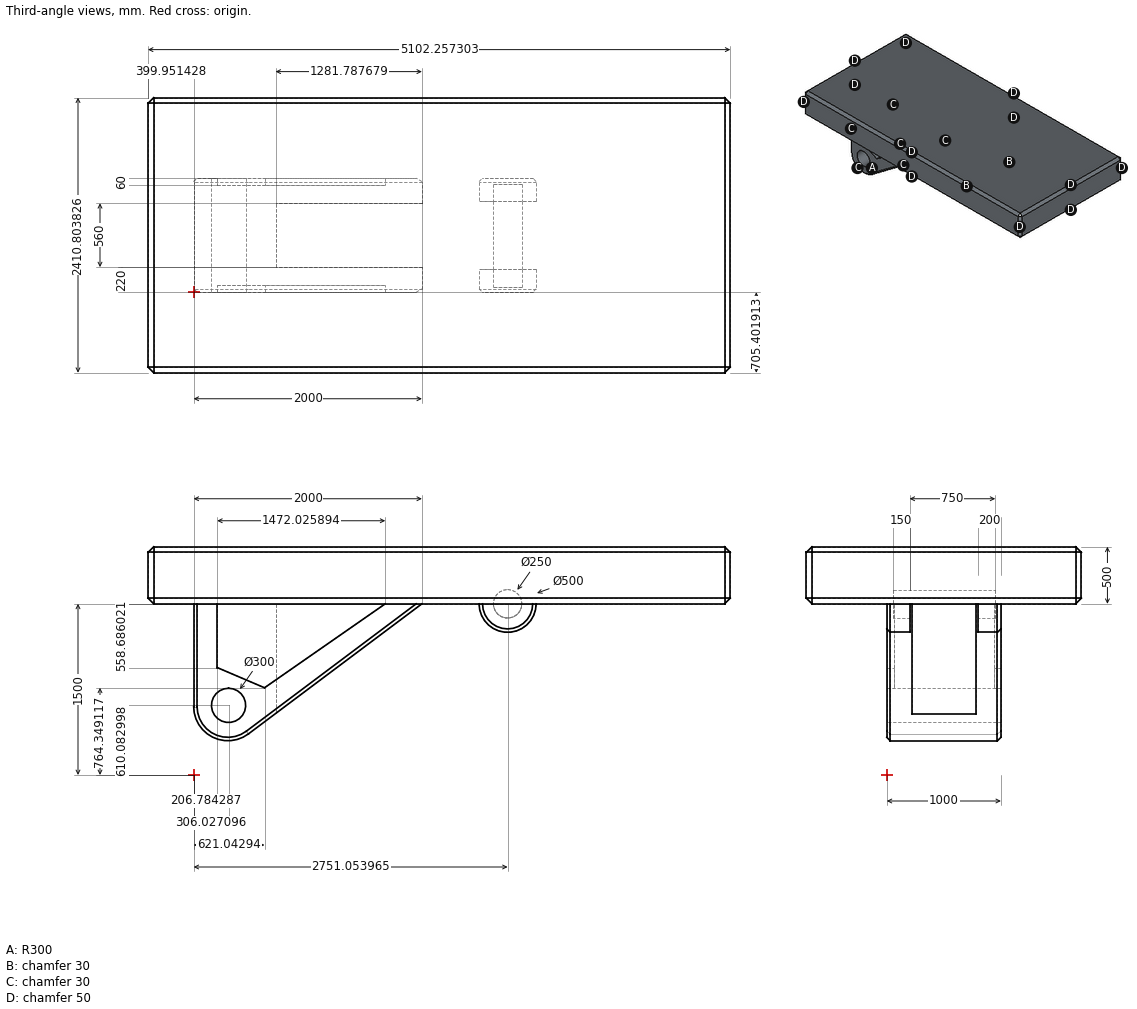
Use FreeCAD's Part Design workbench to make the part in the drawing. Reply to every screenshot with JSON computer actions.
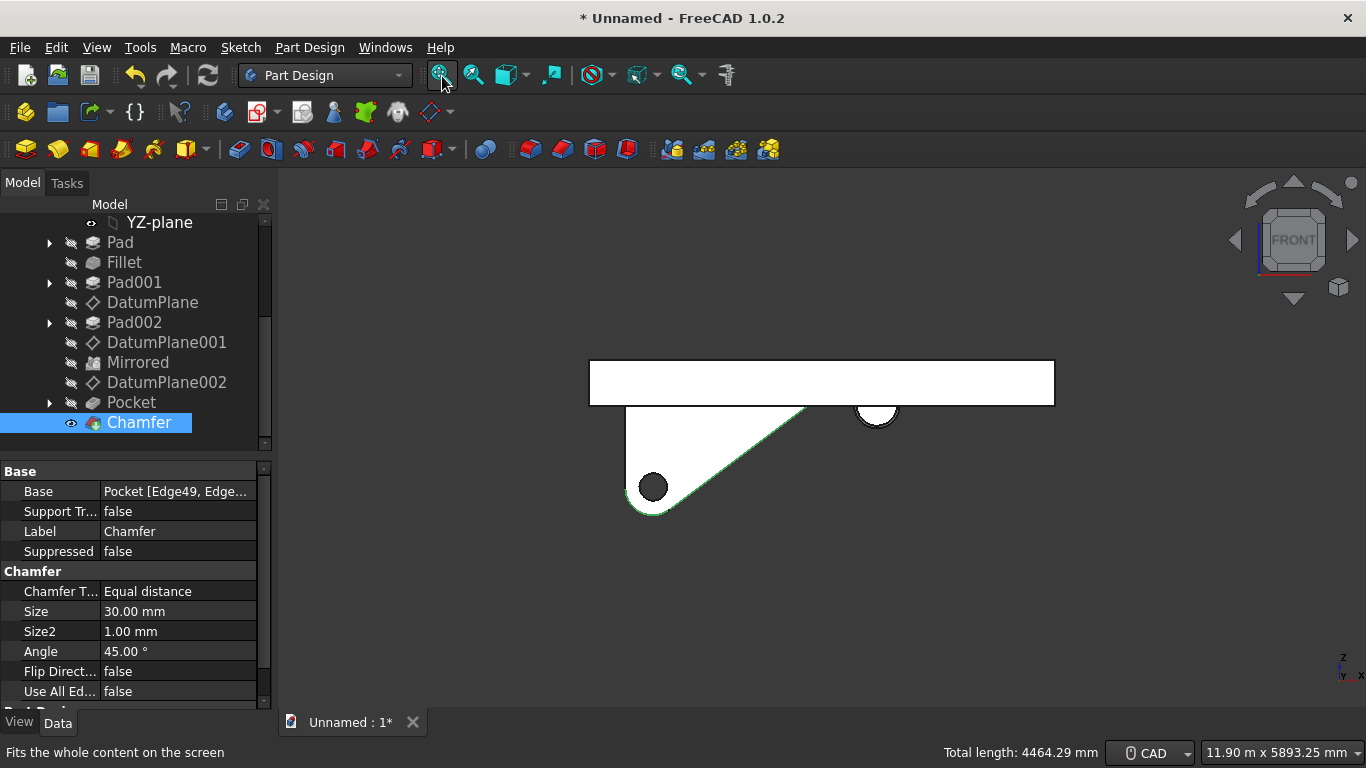
{"action": "left_click", "coordinate": [442, 76]}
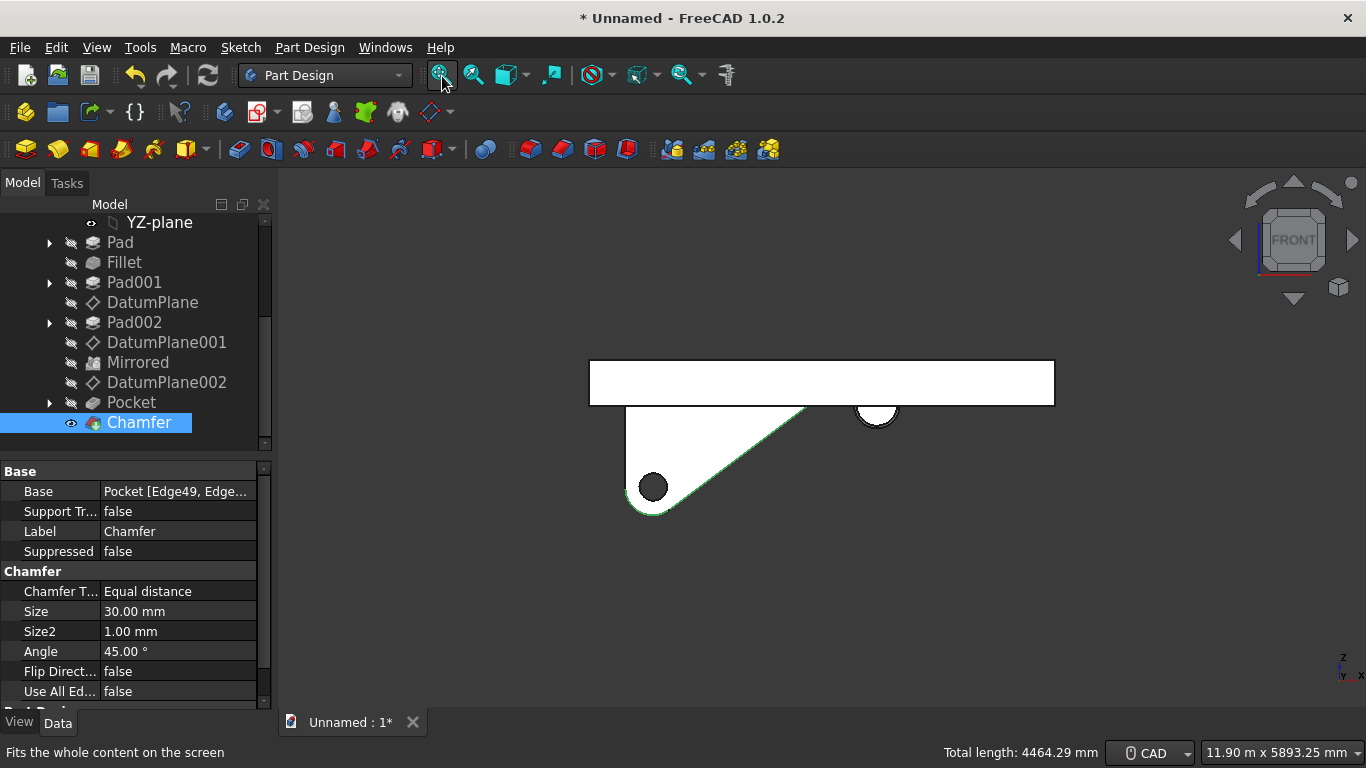
{"action": "left_click", "coordinate": [625, 446], "text": "ctrl"}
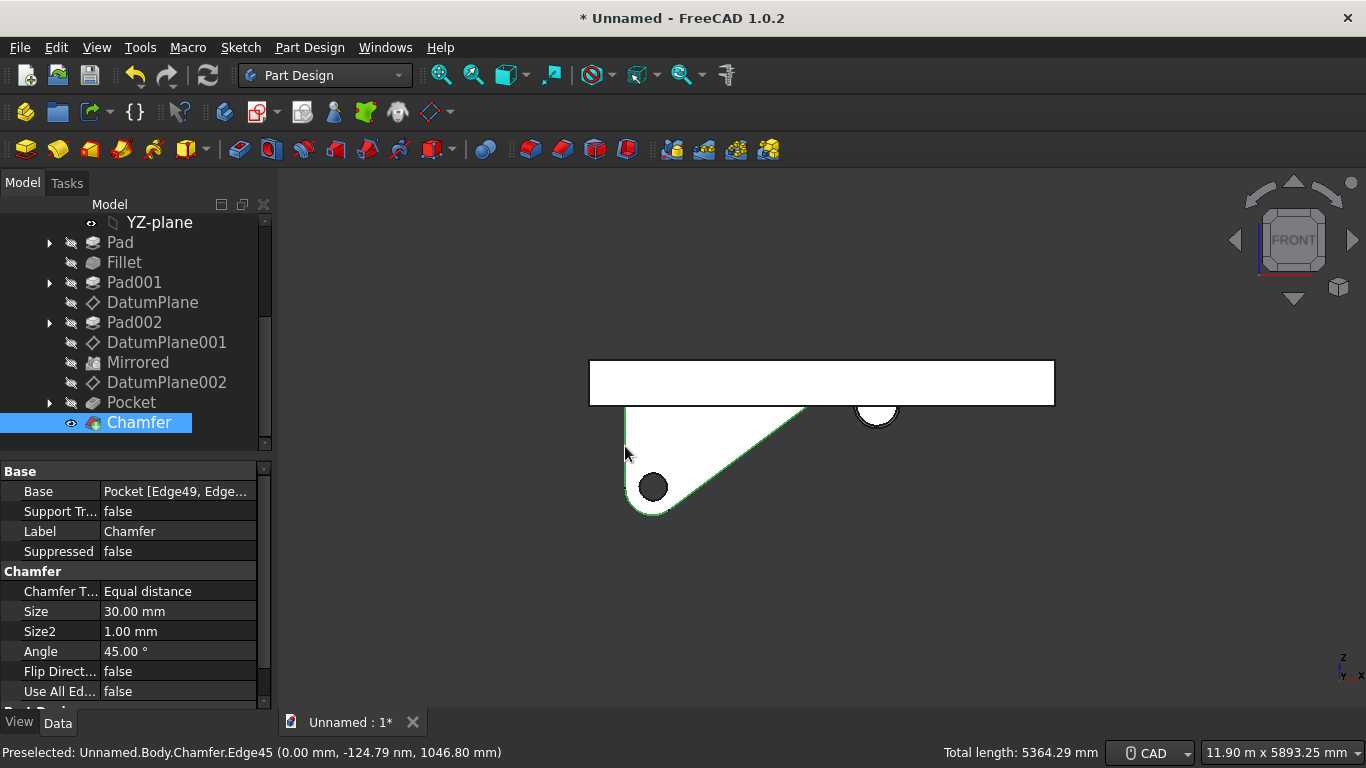
{"action": "key", "text": "3"}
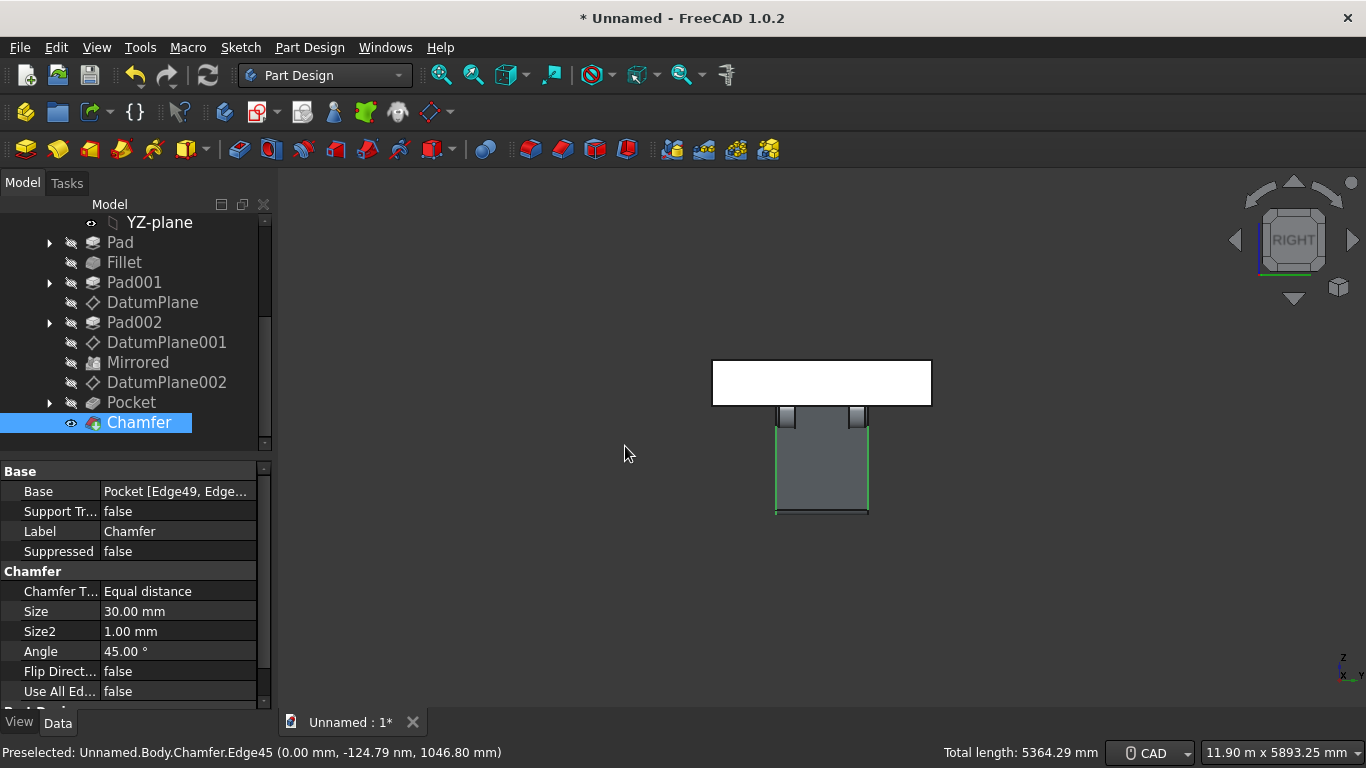
{"action": "left_click", "coordinate": [442, 76]}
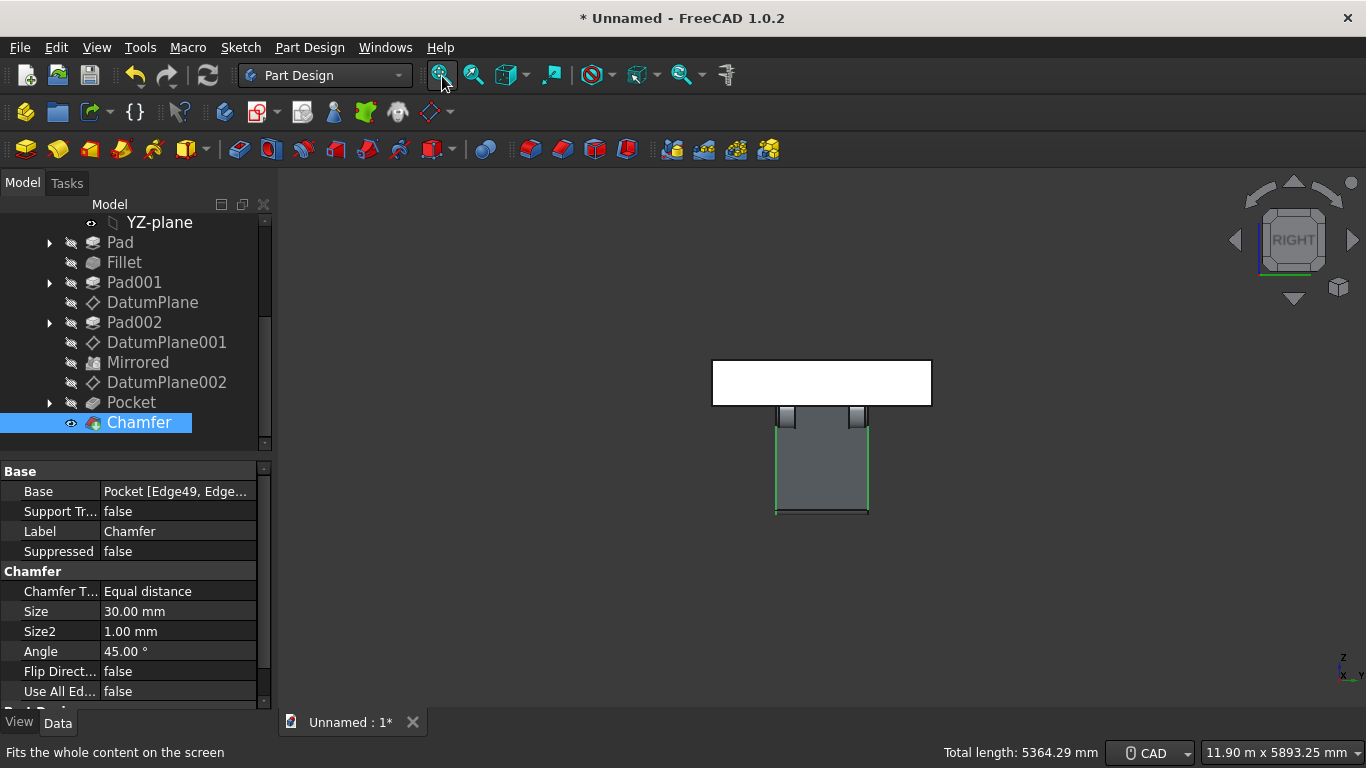
{"action": "key", "text": "5"}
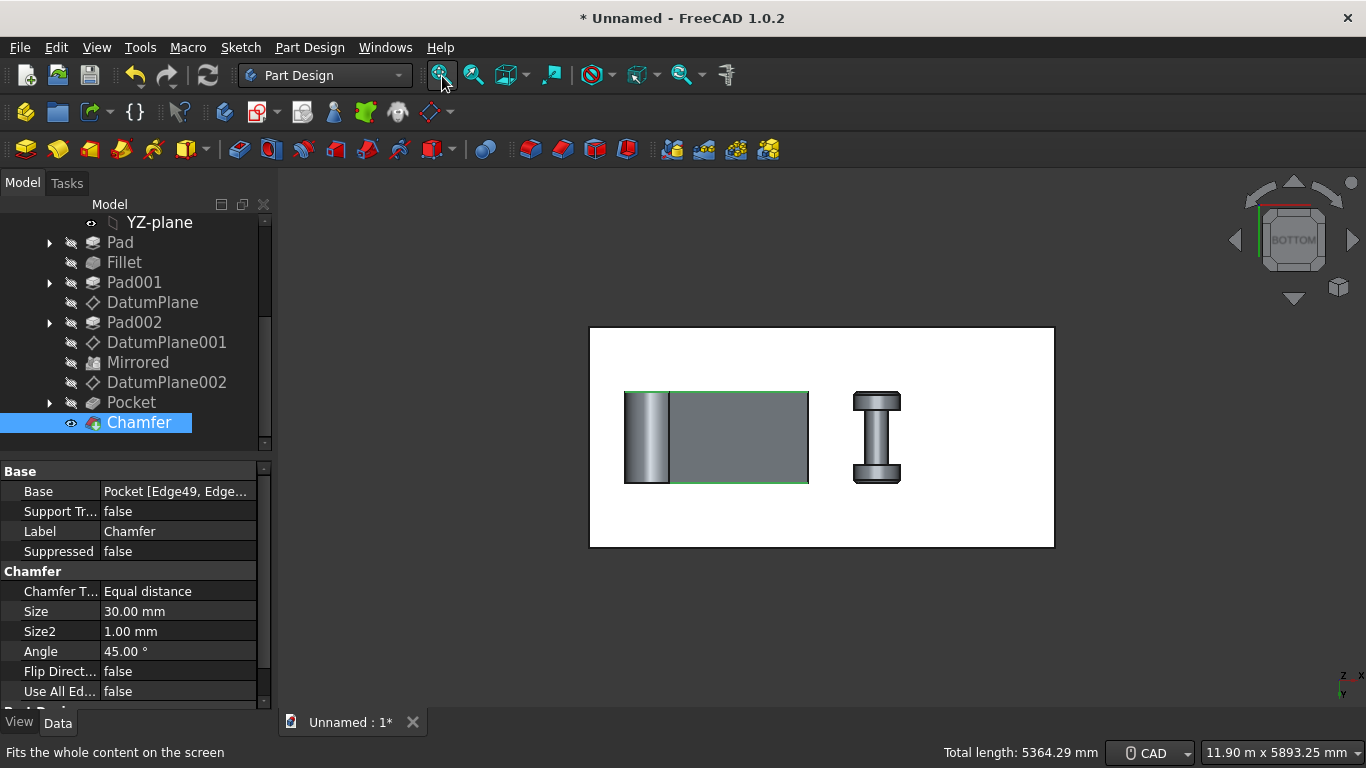
{"action": "key", "text": "v f"}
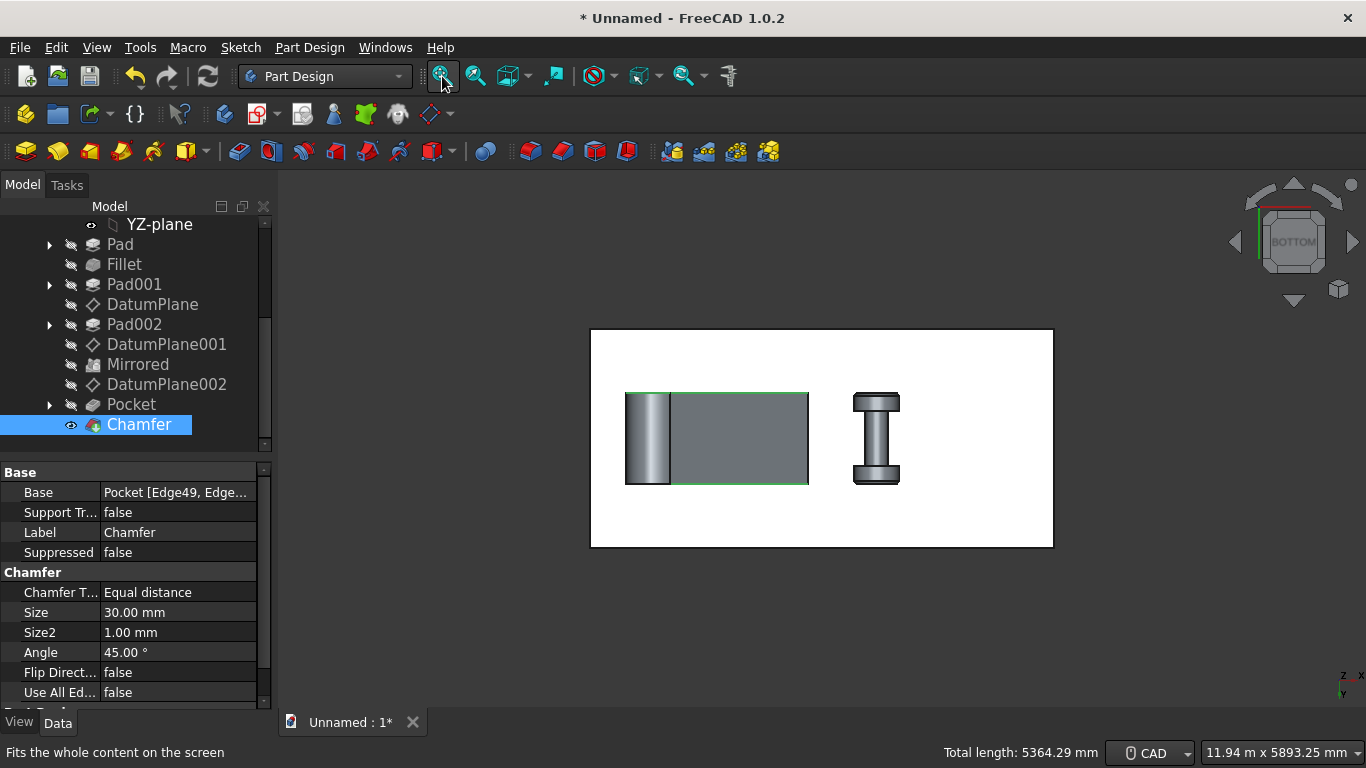
{"action": "left_click", "coordinate": [641, 483], "text": "ctrl"}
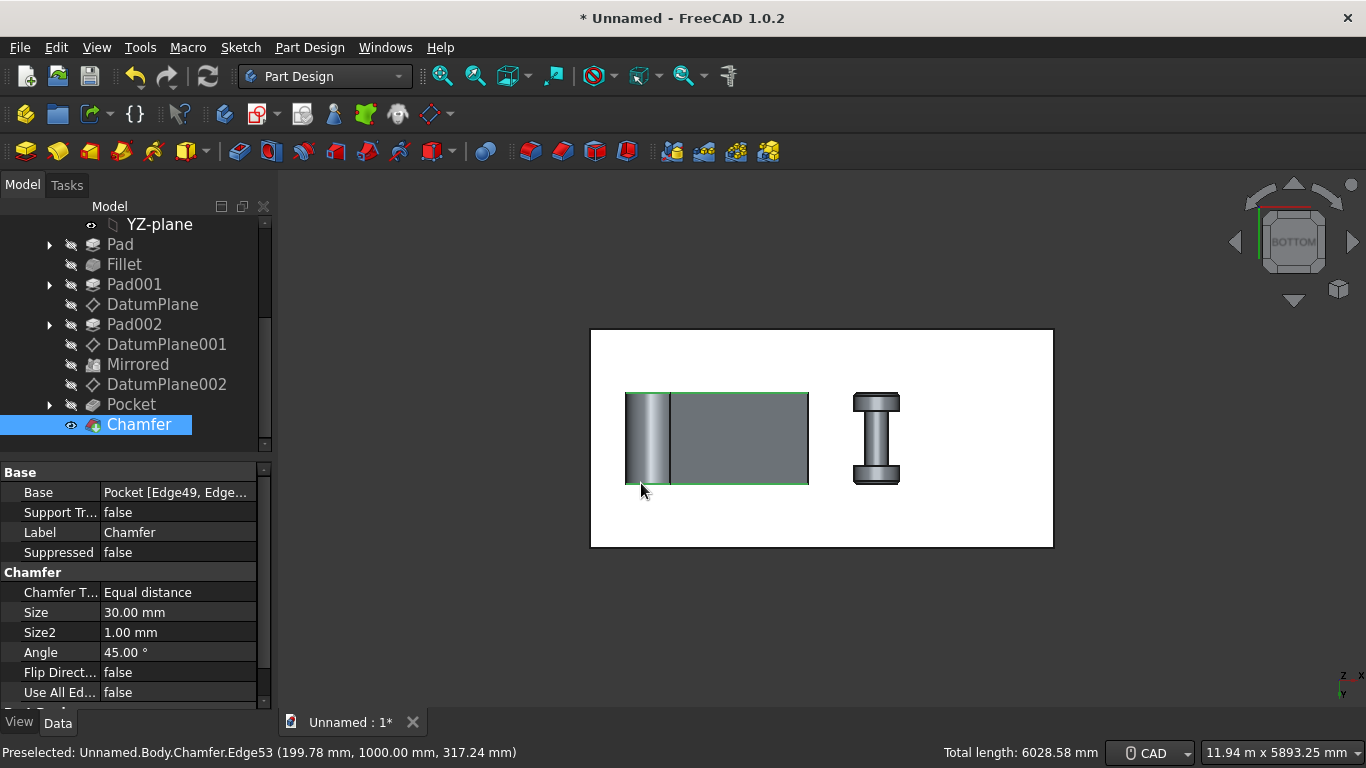
{"action": "key", "text": "4"}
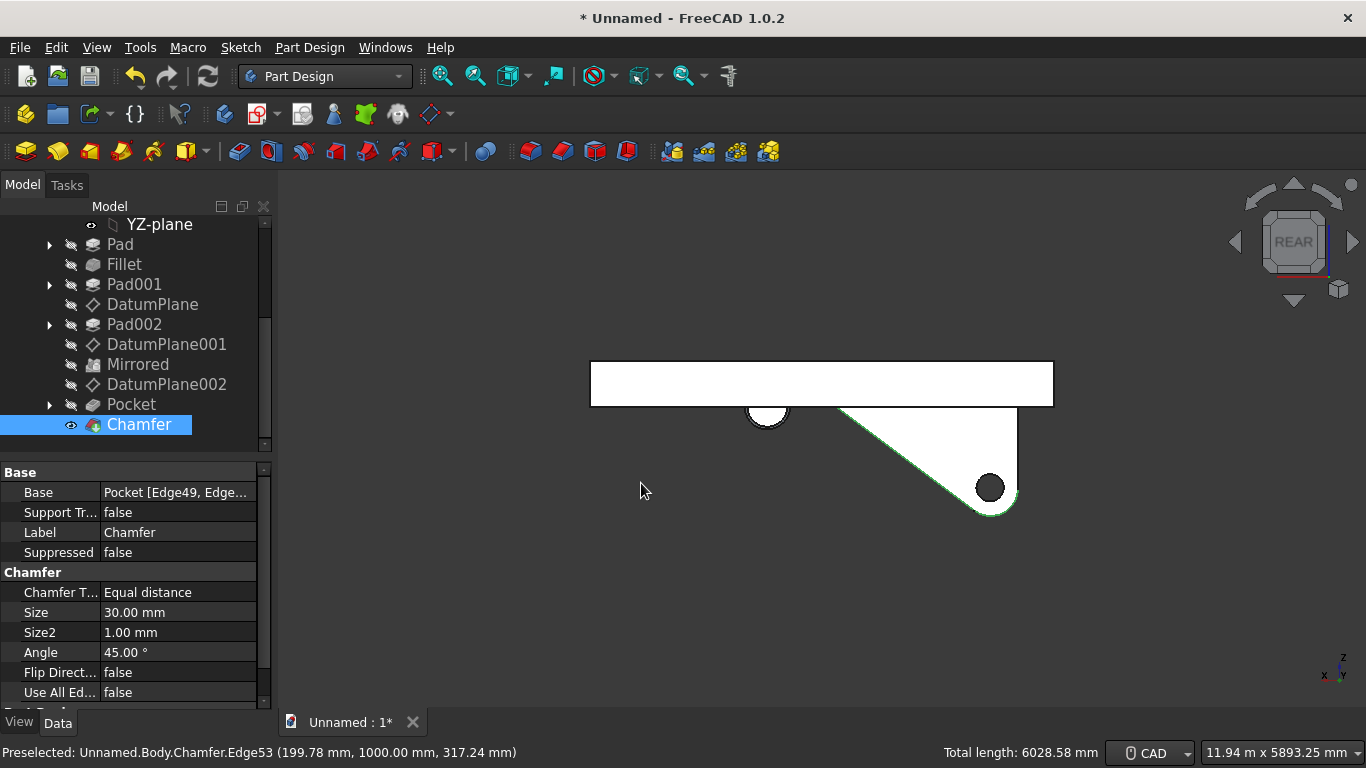
{"action": "left_click", "coordinate": [444, 76]}